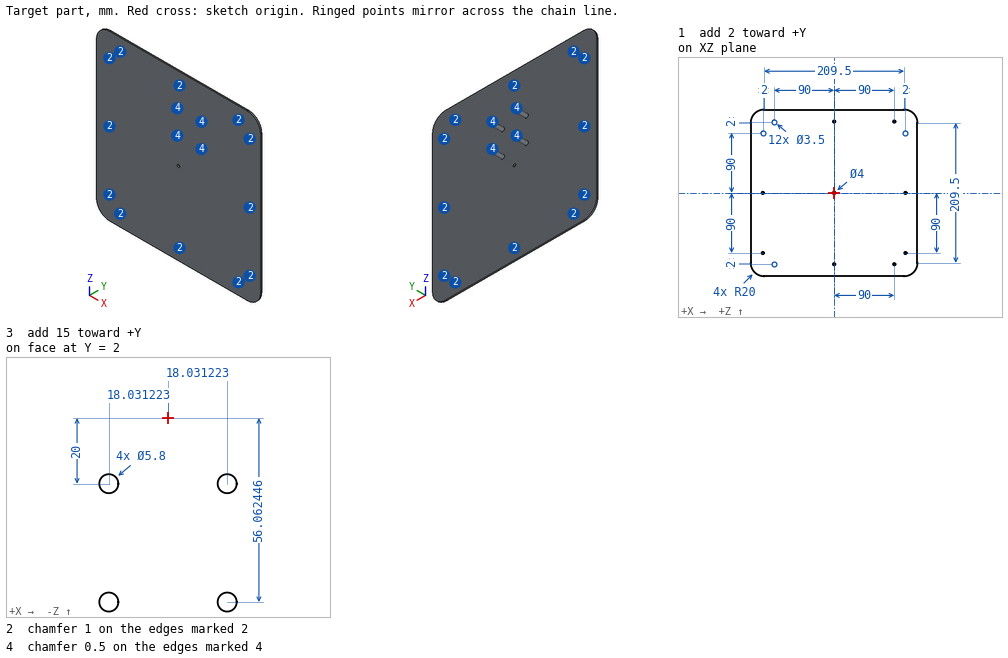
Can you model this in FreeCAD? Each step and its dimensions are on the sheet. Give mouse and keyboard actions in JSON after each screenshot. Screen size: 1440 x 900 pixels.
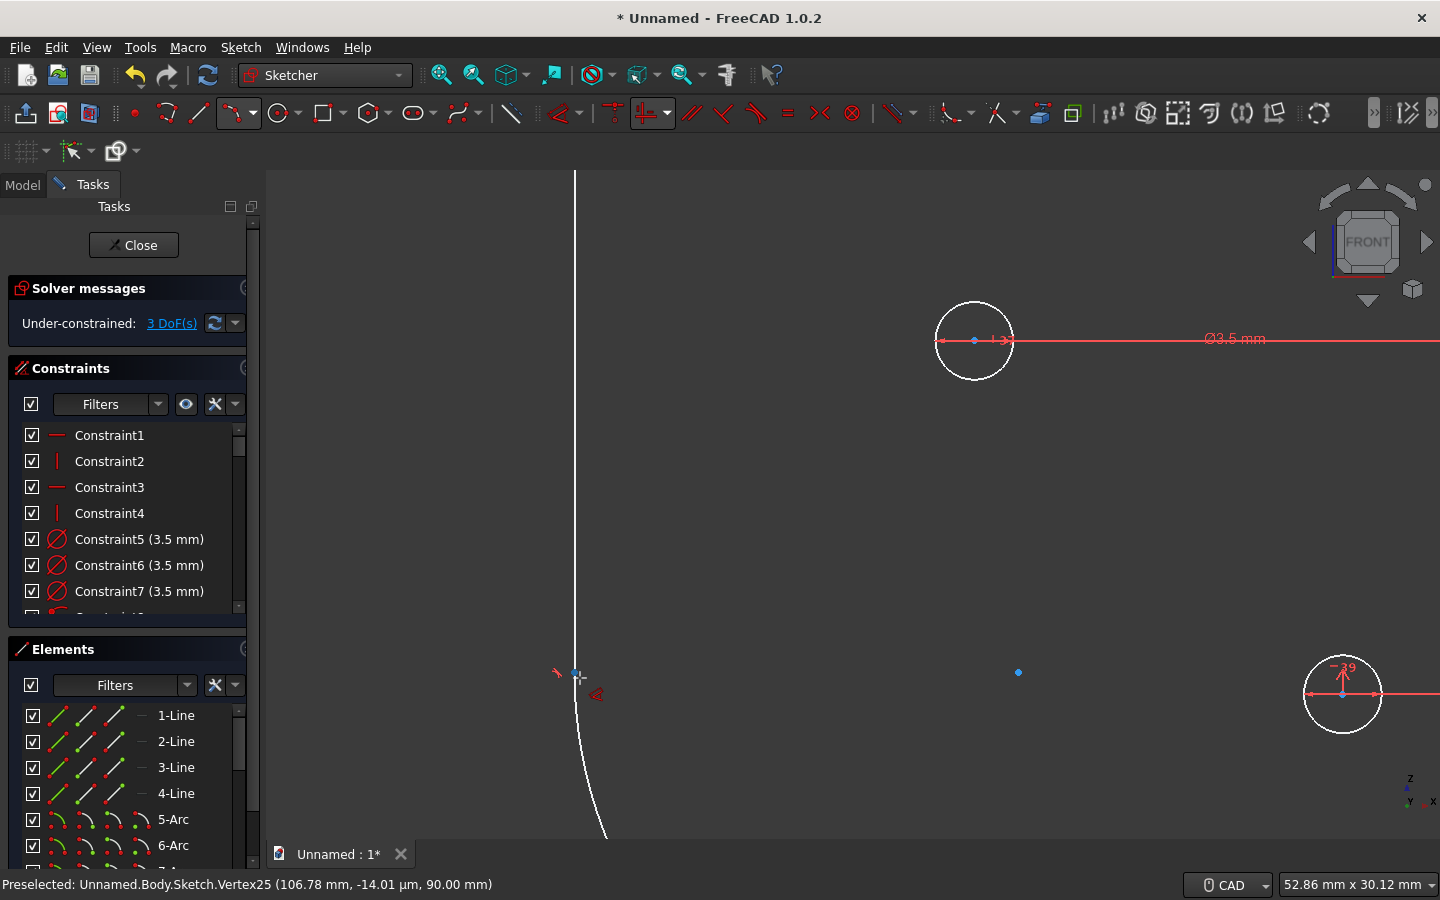
{"action": "left_click", "coordinate": [575, 673]}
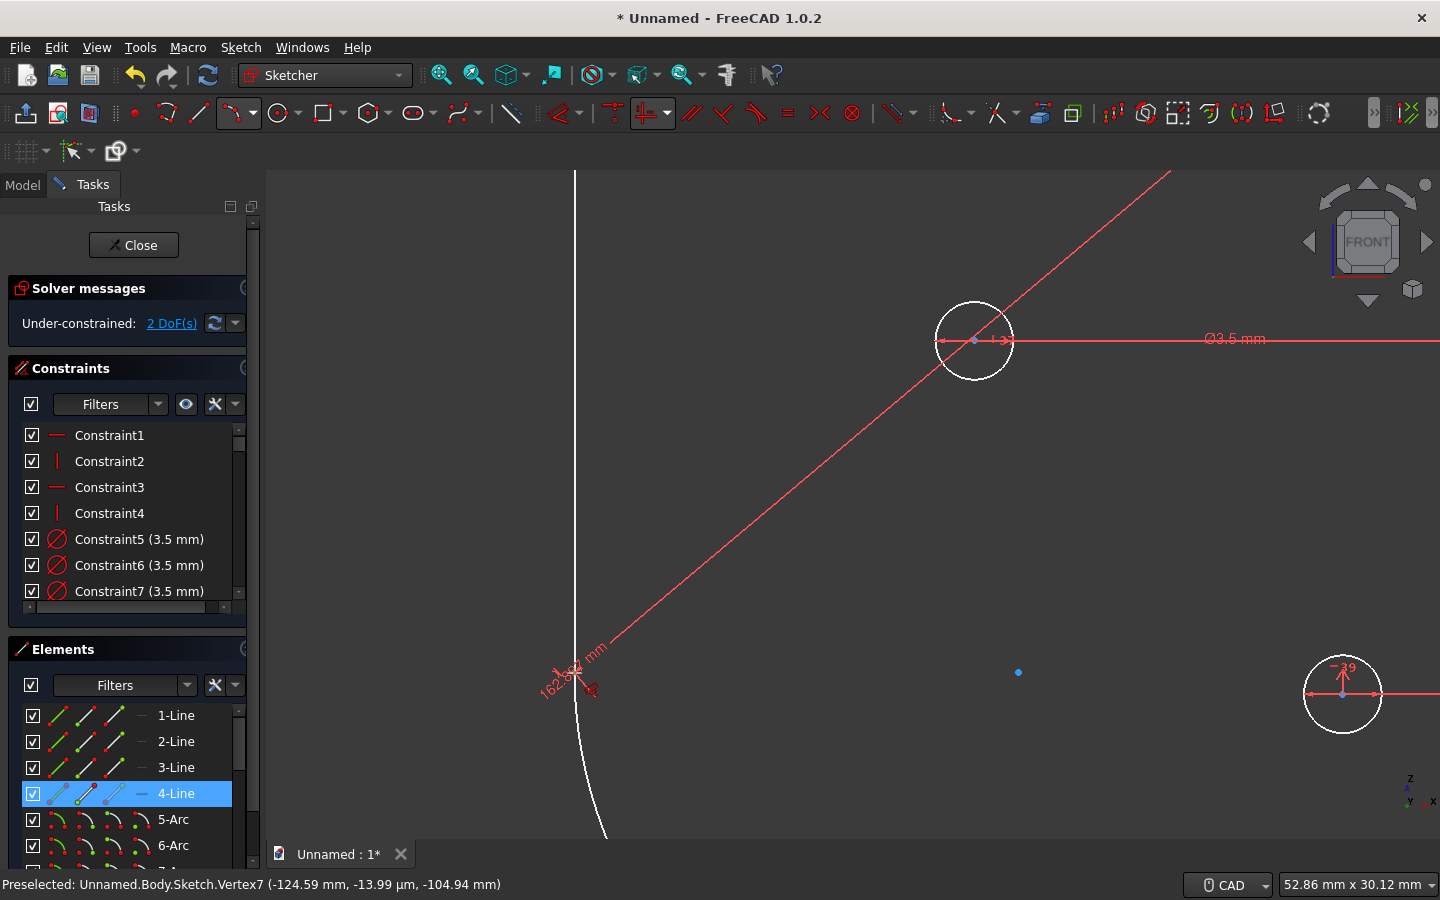
{"action": "scroll", "coordinate": [579, 678], "scroll_direction": "down", "scroll_amount": 13}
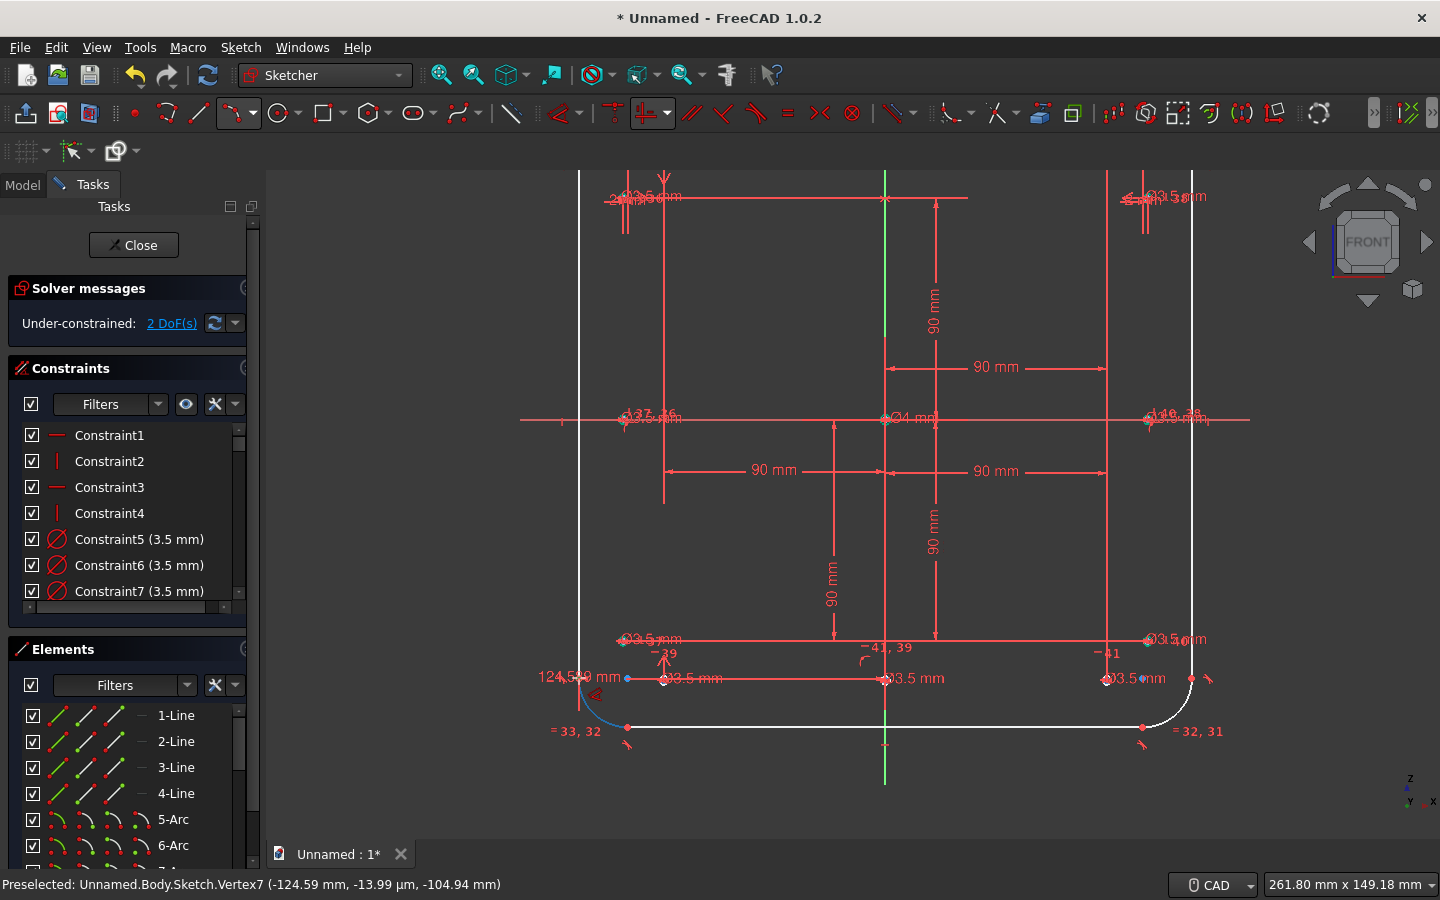
{"action": "scroll", "coordinate": [636, 680], "scroll_direction": "up", "scroll_amount": 13}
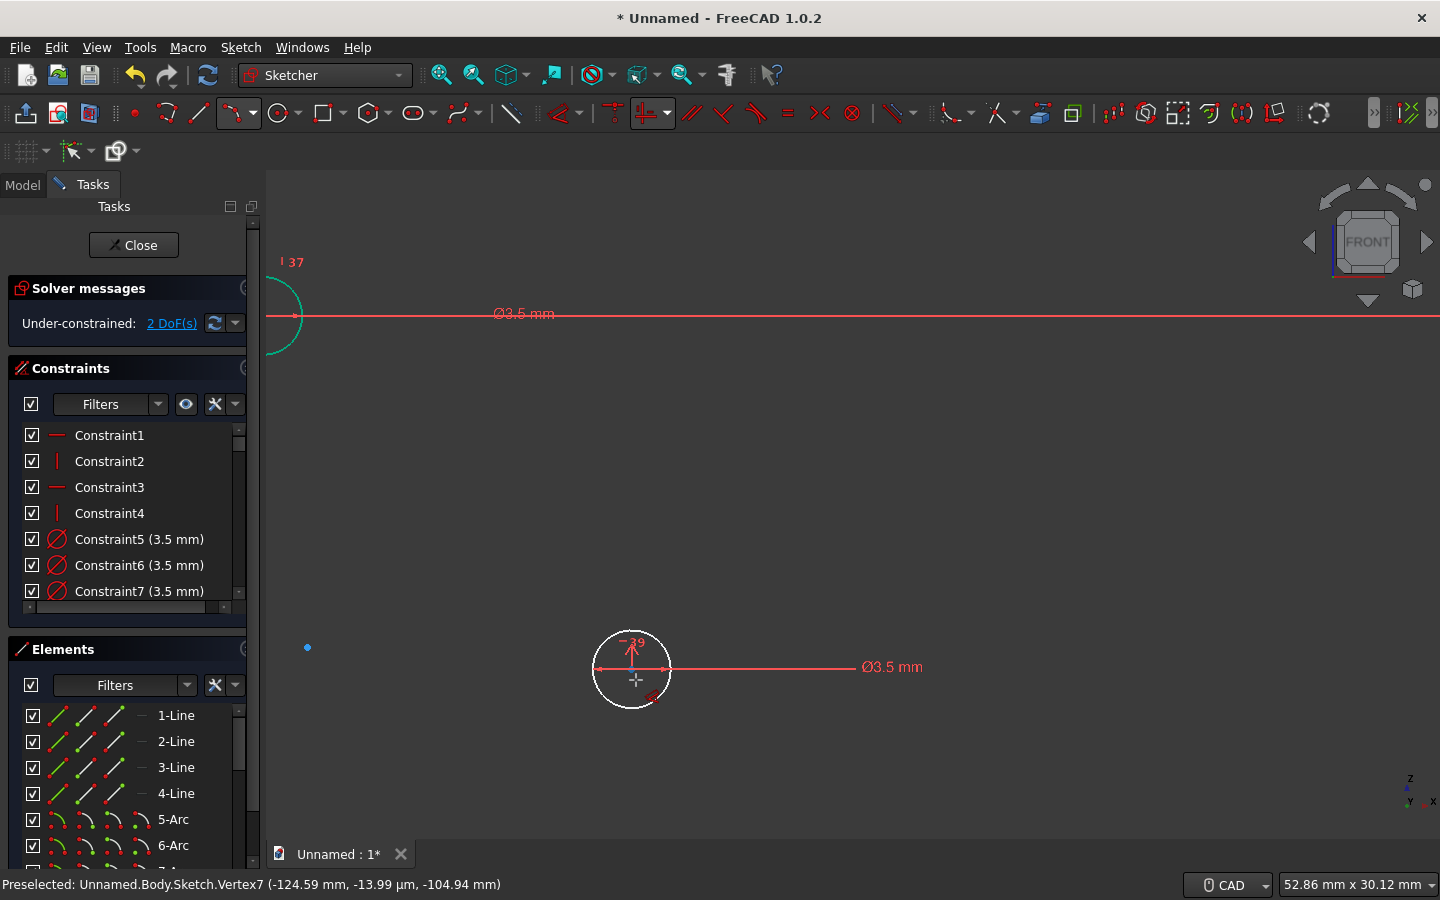
{"action": "left_click", "coordinate": [632, 669]}
{"action": "left_click", "coordinate": [690, 659]}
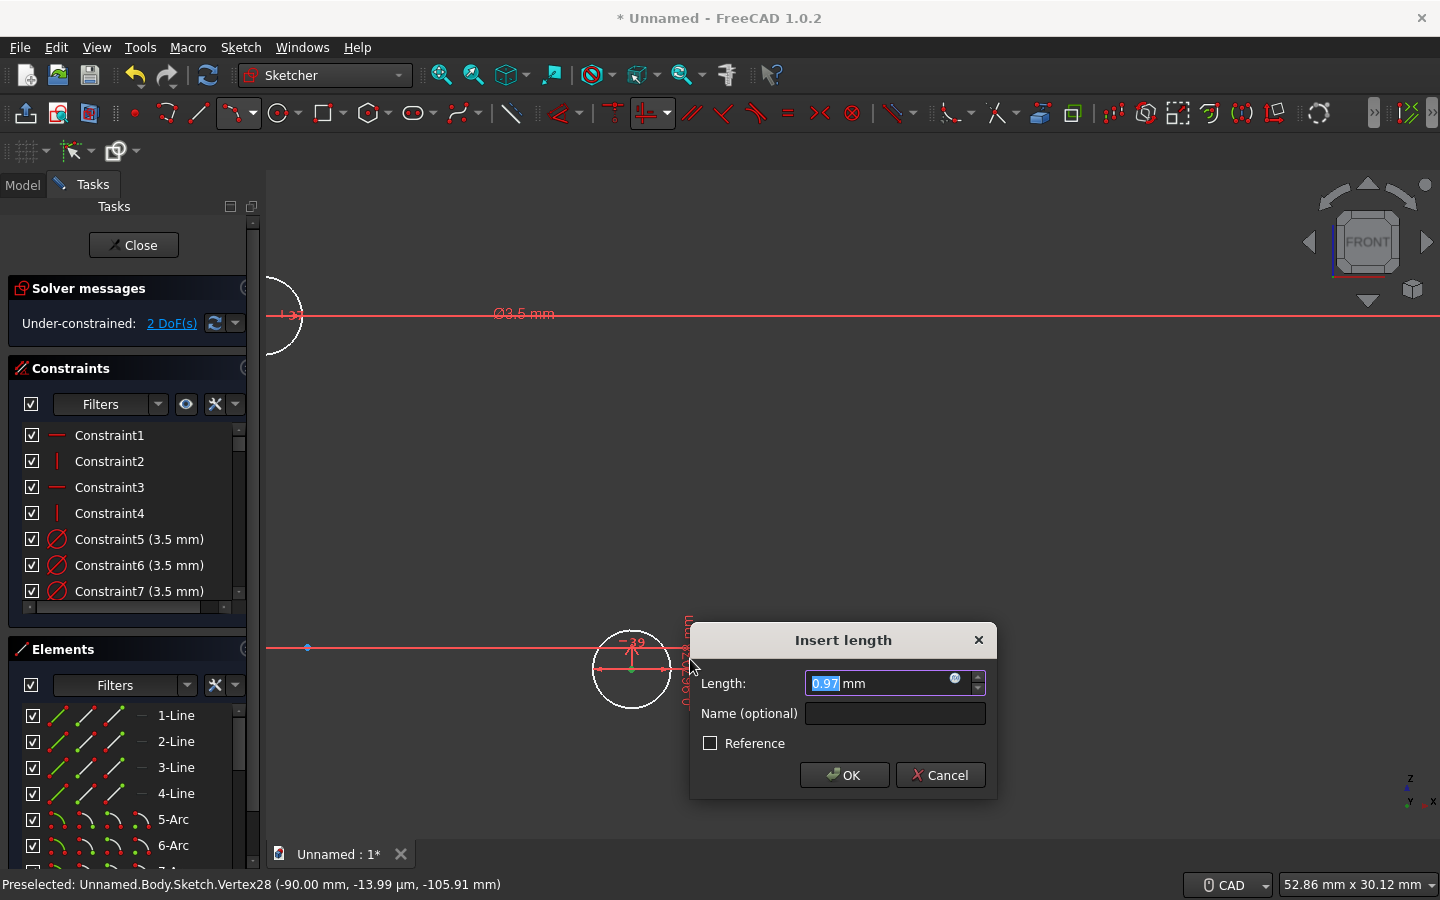
{"action": "type", "text": "2"}
{"action": "key", "text": "Return"}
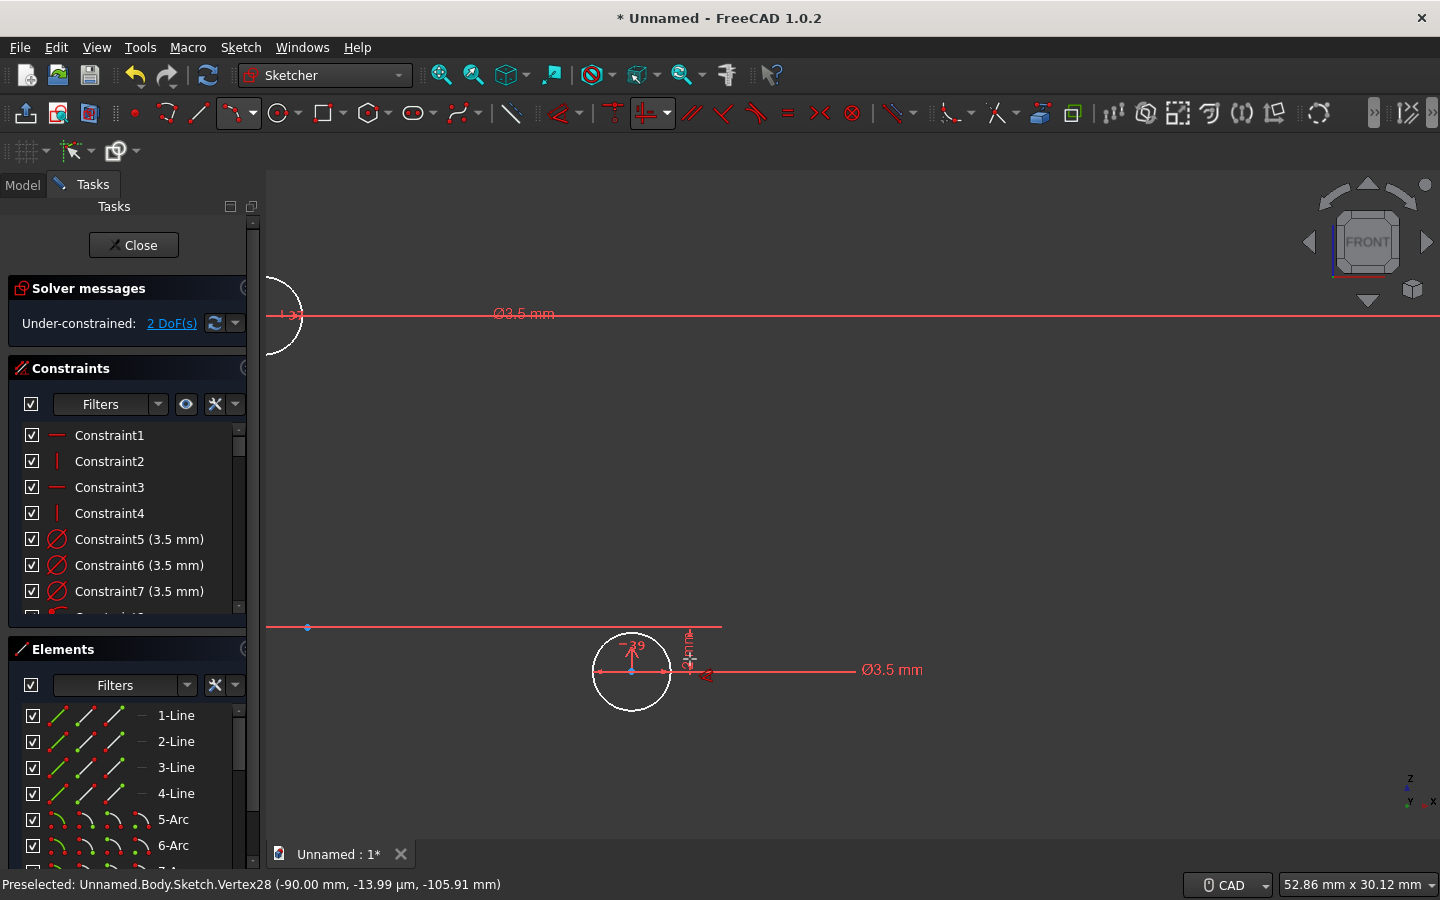
{"action": "scroll", "coordinate": [636, 680], "scroll_direction": "down", "scroll_amount": 13}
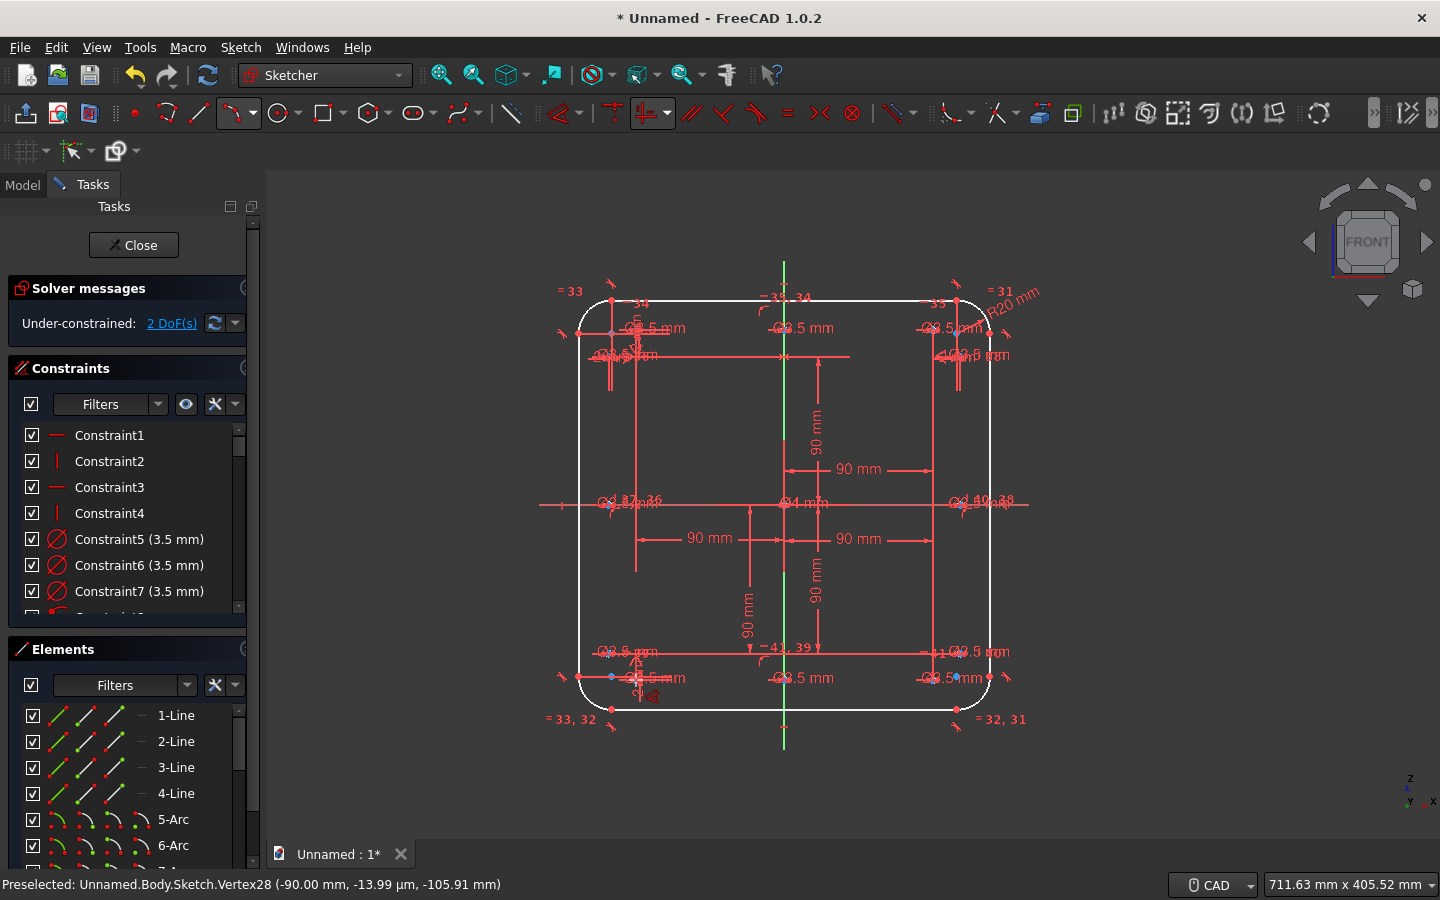
{"action": "left_click", "coordinate": [715, 301]}
{"action": "left_click", "coordinate": [705, 267]}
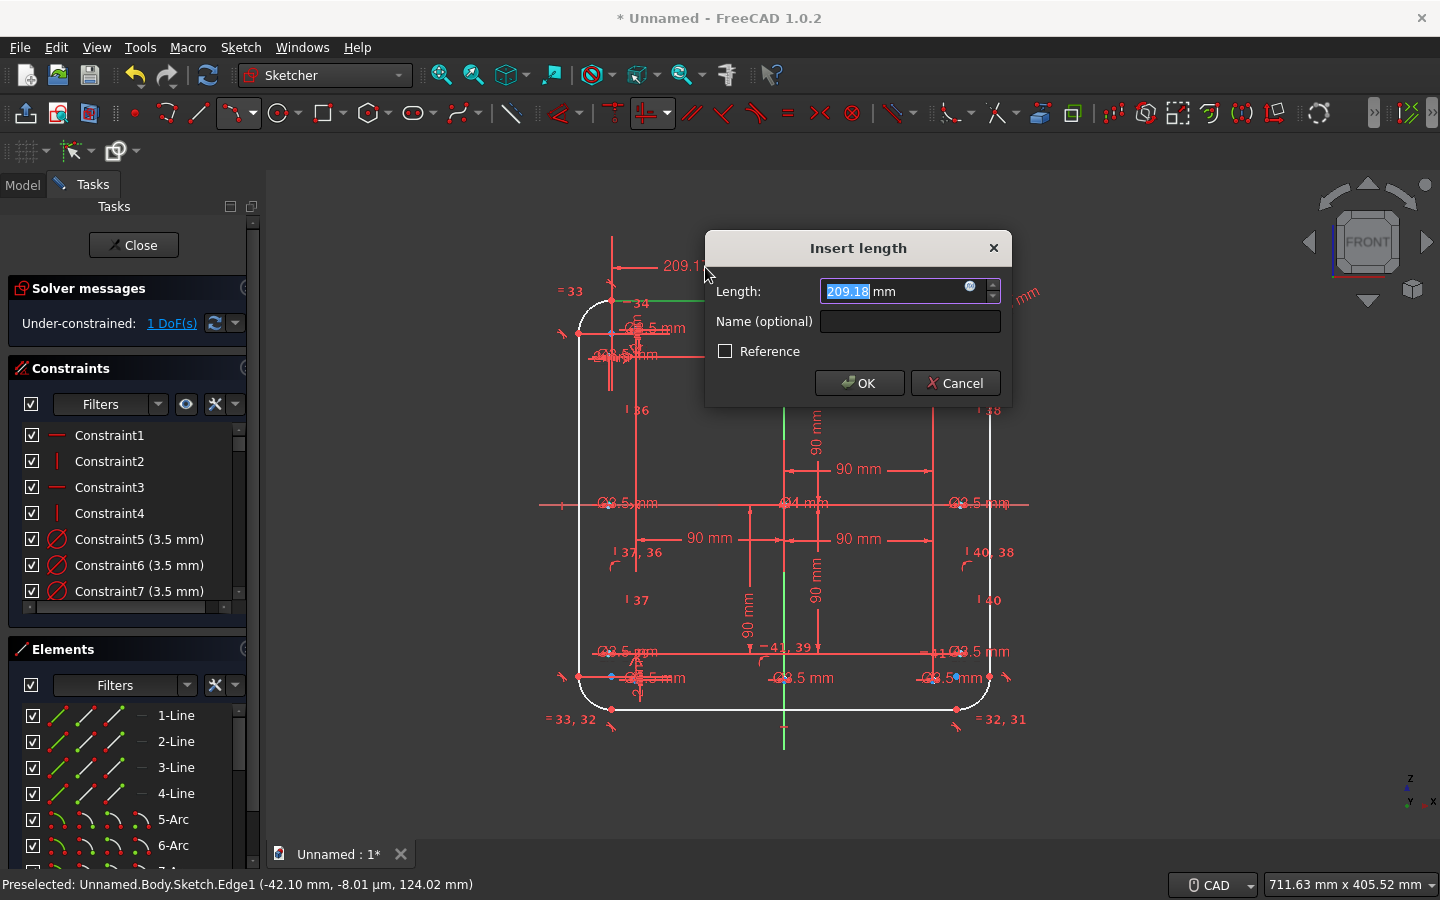
{"action": "type", "text": "209.5"}
{"action": "key", "text": "Return"}